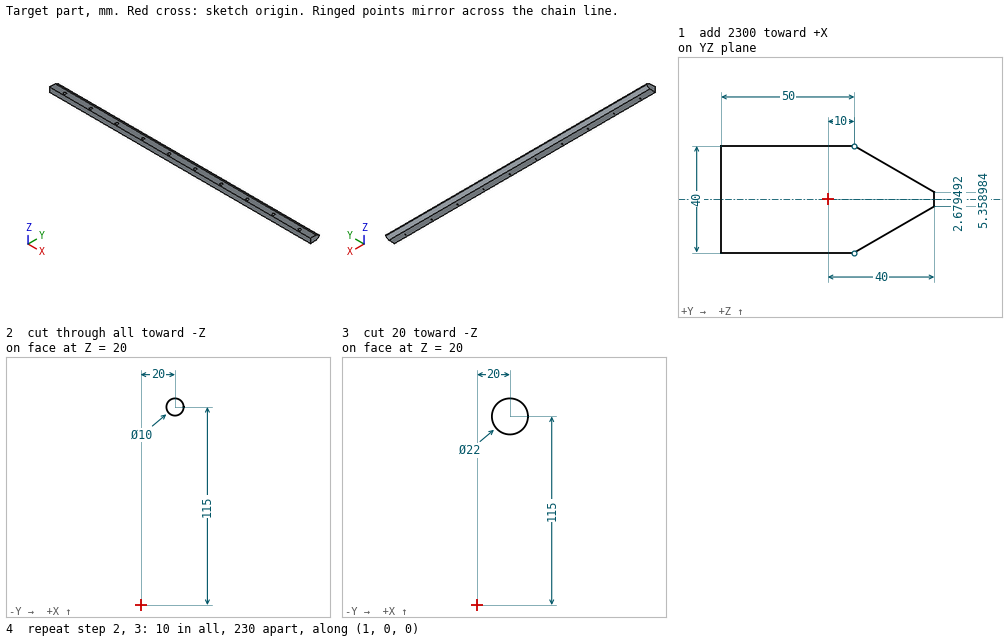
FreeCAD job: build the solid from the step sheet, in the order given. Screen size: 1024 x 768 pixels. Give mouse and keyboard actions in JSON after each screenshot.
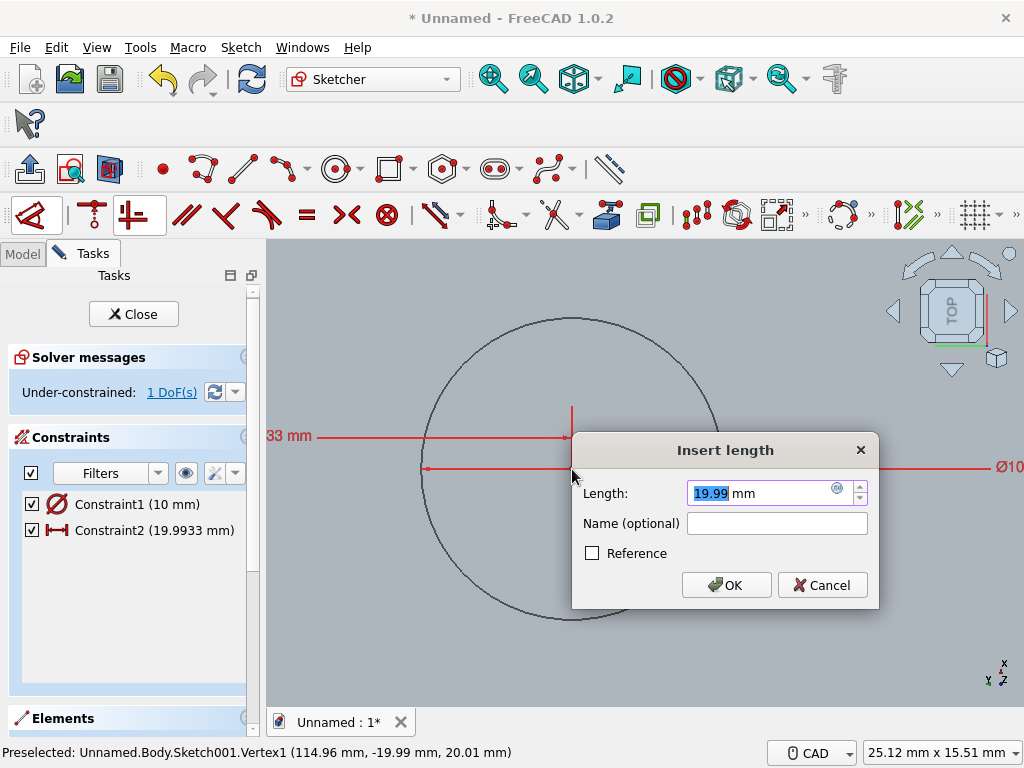
{"action": "type", "text": "20"}
{"action": "key", "text": "Return"}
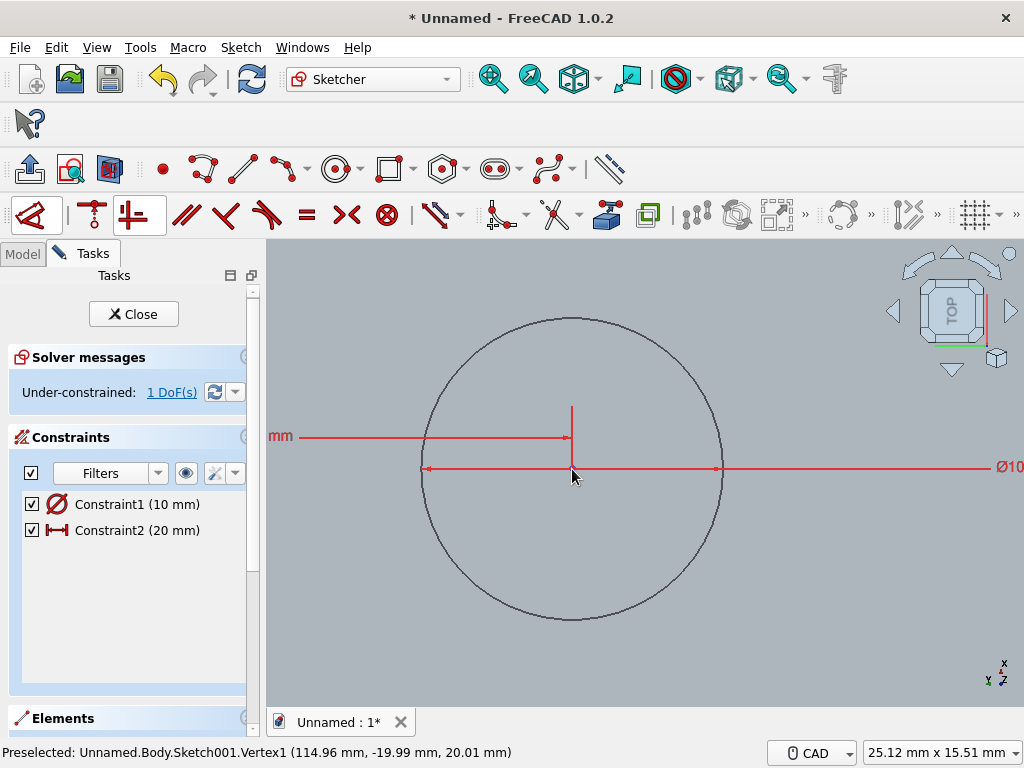
{"action": "left_click", "coordinate": [572, 469]}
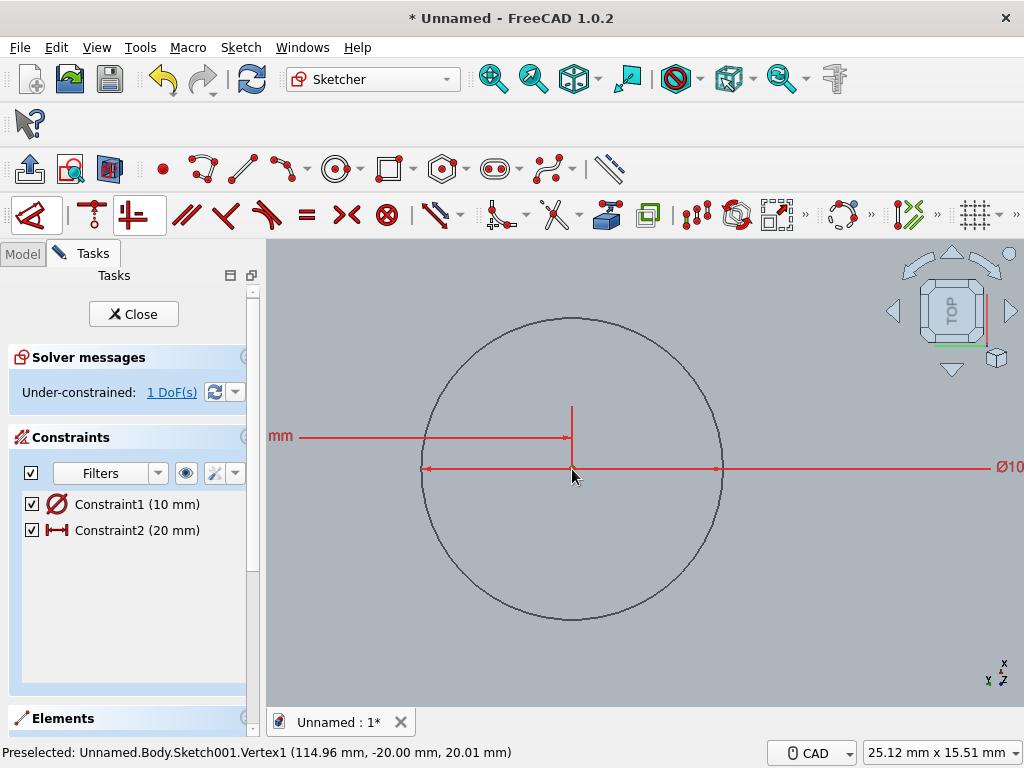
{"action": "key", "text": "i"}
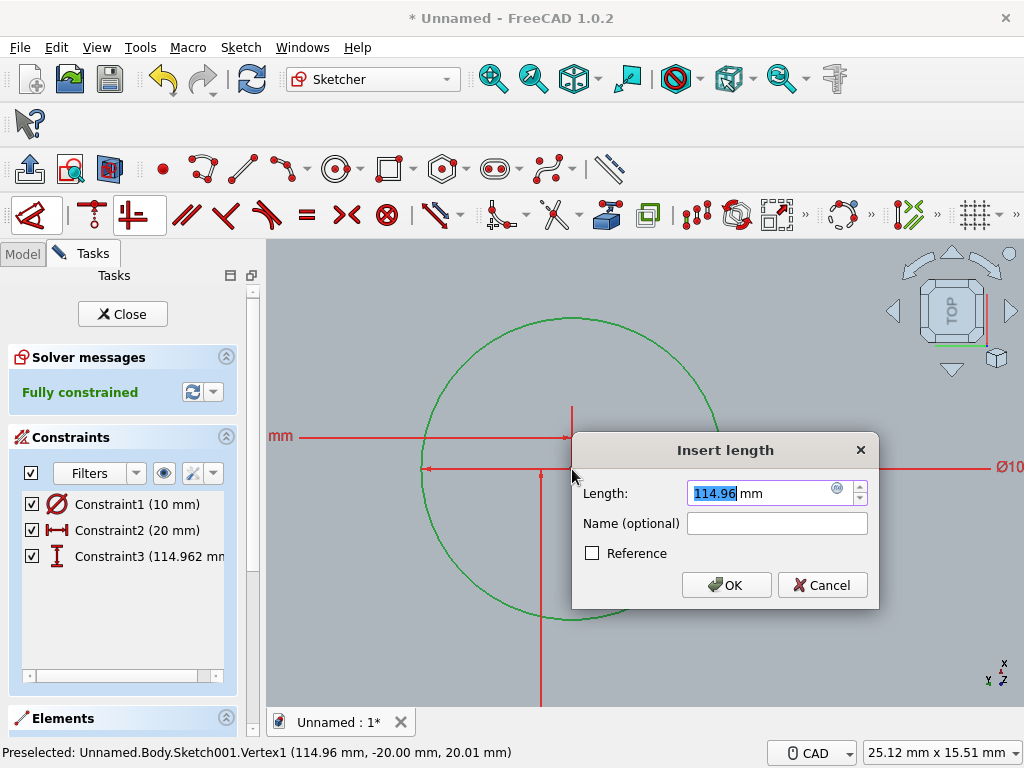
{"action": "type", "text": "115"}
{"action": "key", "text": "Return"}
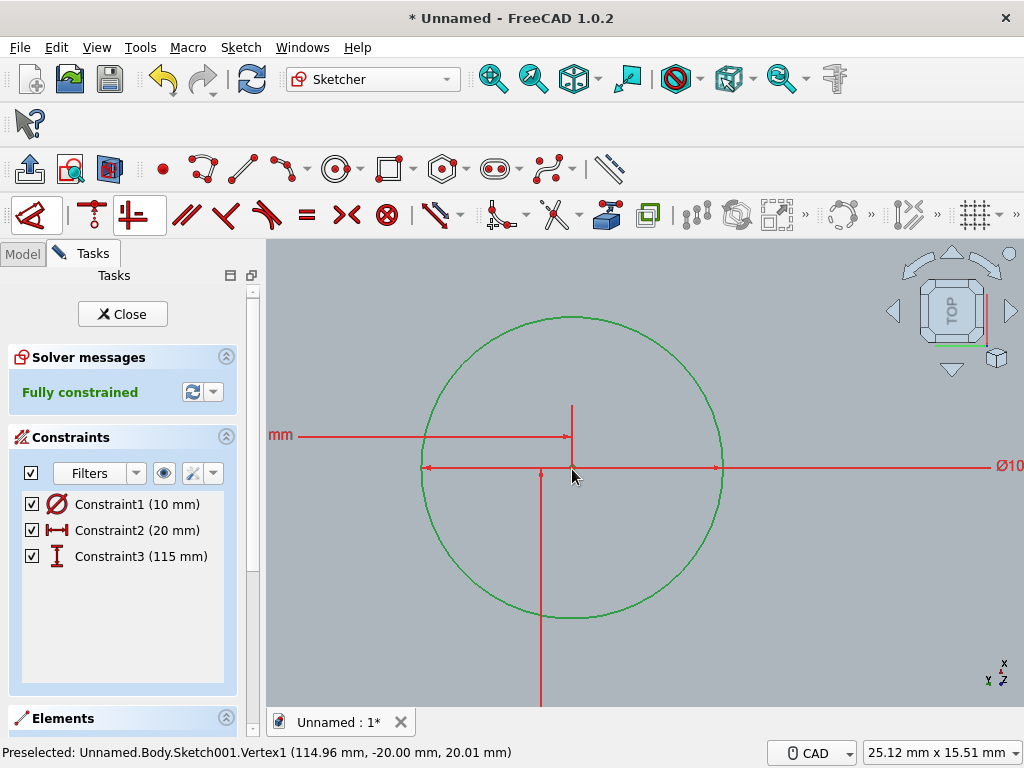
{"action": "left_click", "coordinate": [123, 314]}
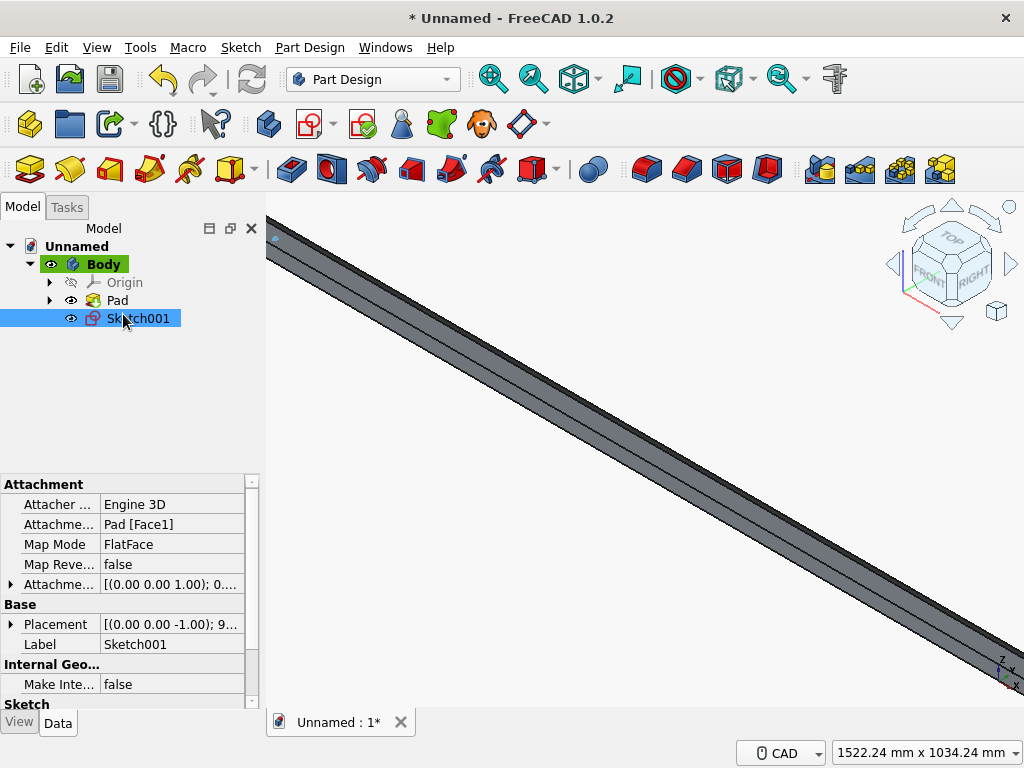
{"action": "left_click", "coordinate": [292, 170]}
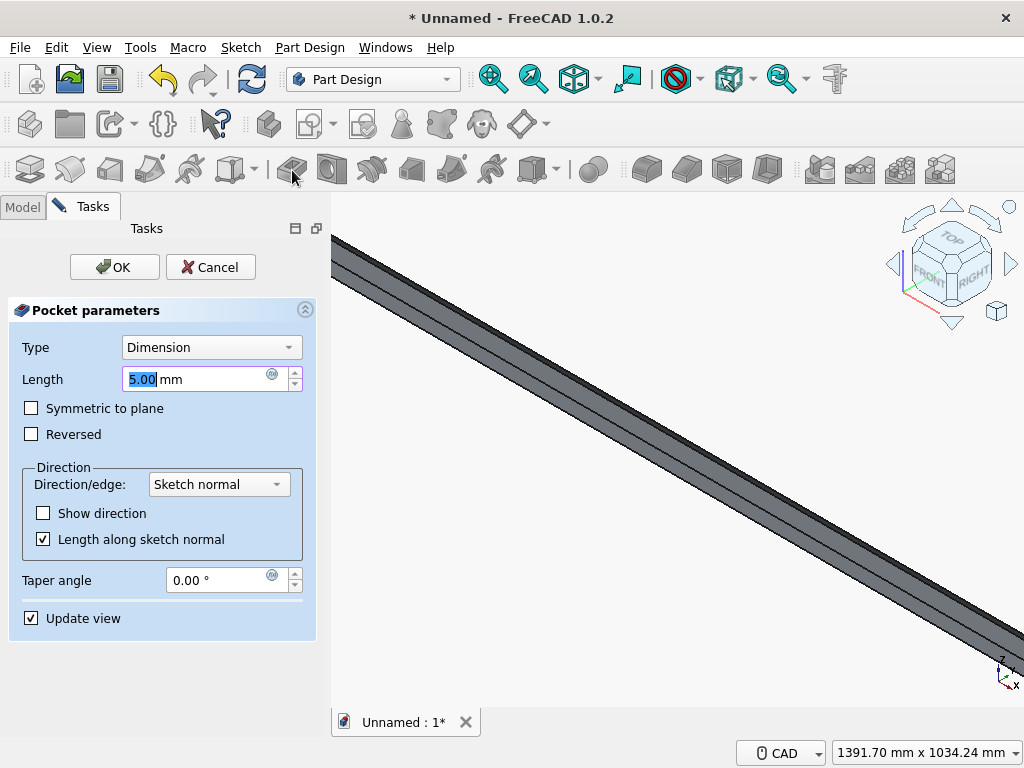
{"action": "left_click", "coordinate": [212, 348]}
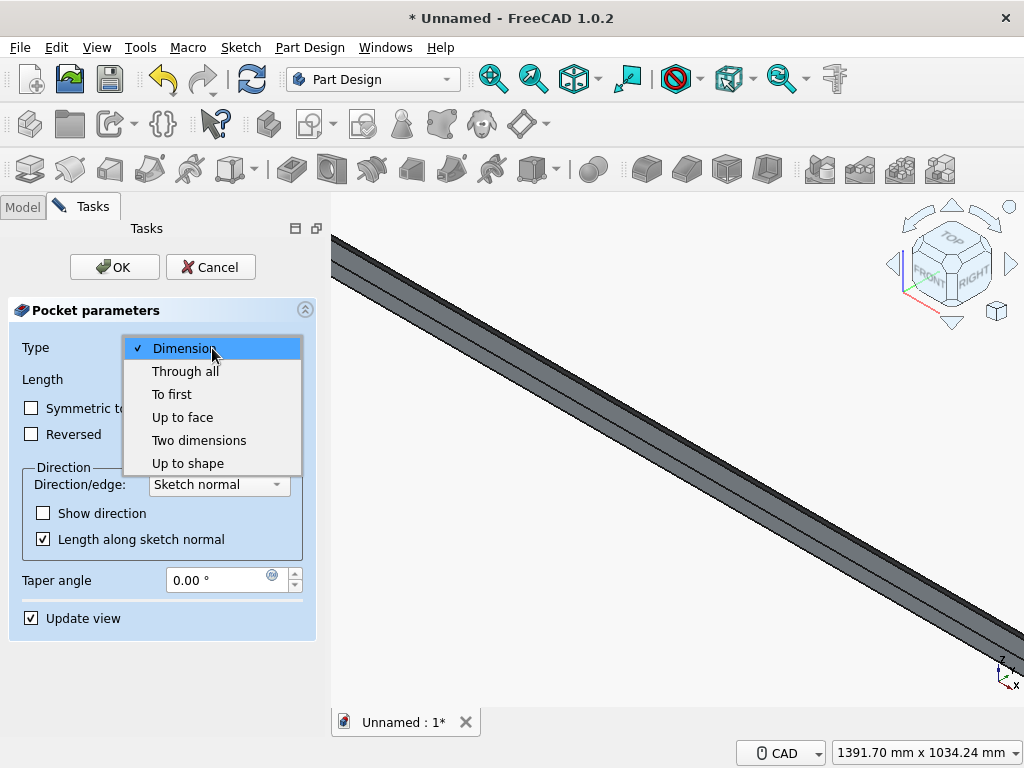
{"action": "left_click", "coordinate": [212, 372]}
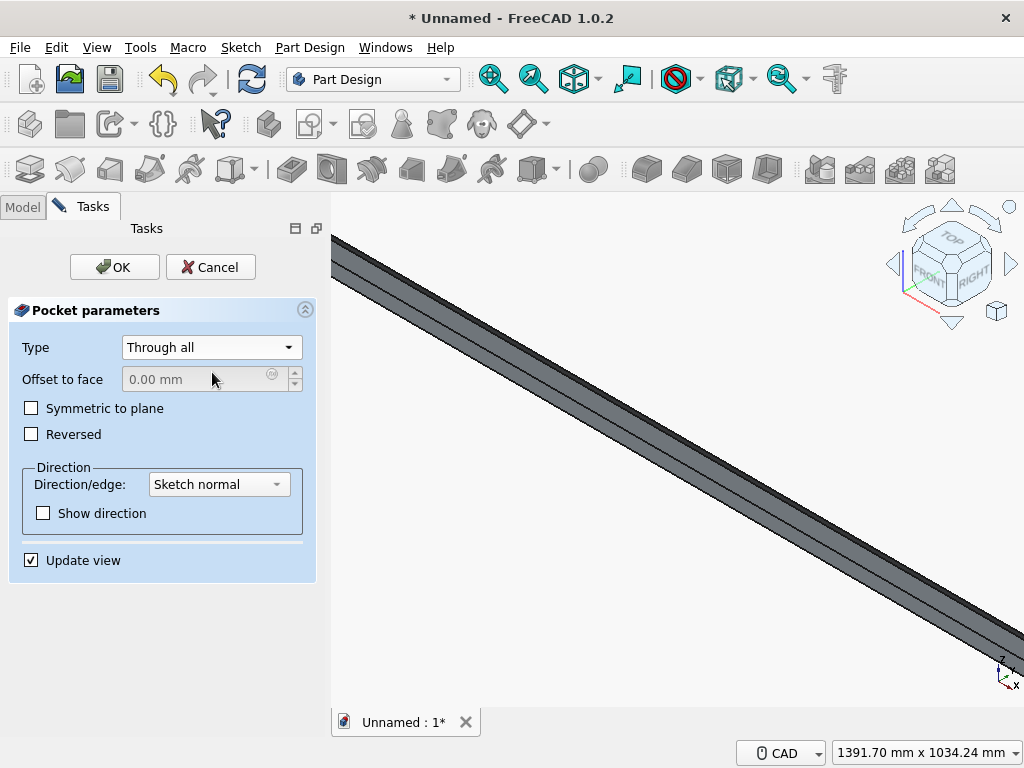
{"action": "left_click", "coordinate": [115, 267]}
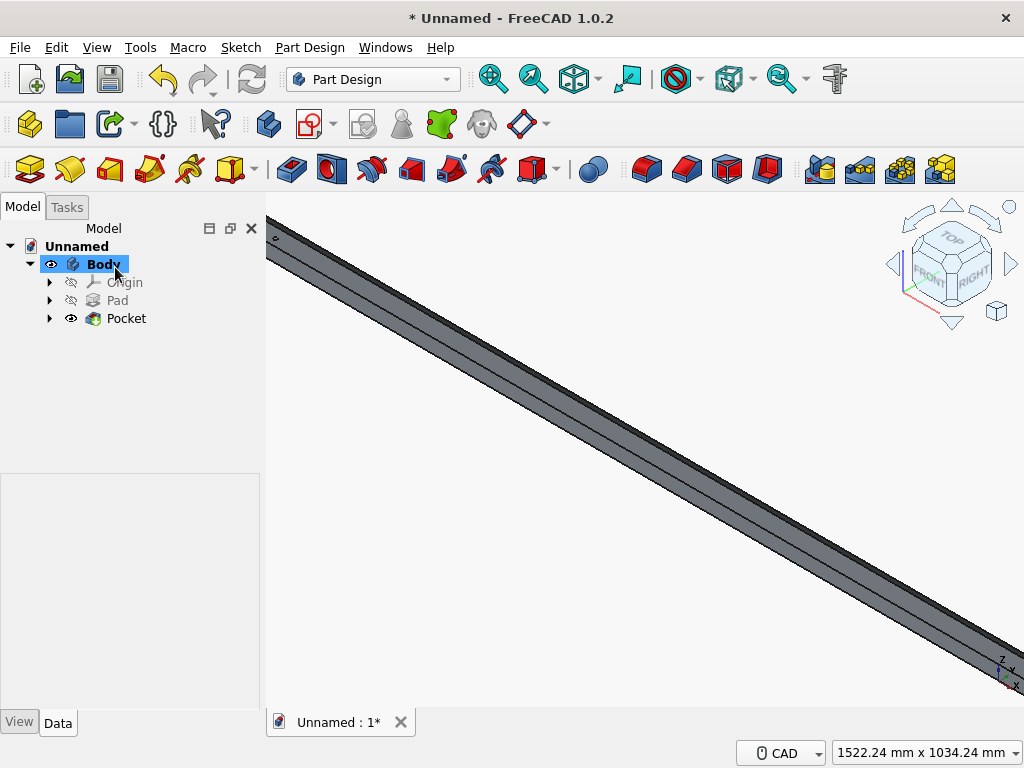
{"action": "key", "text": "v f"}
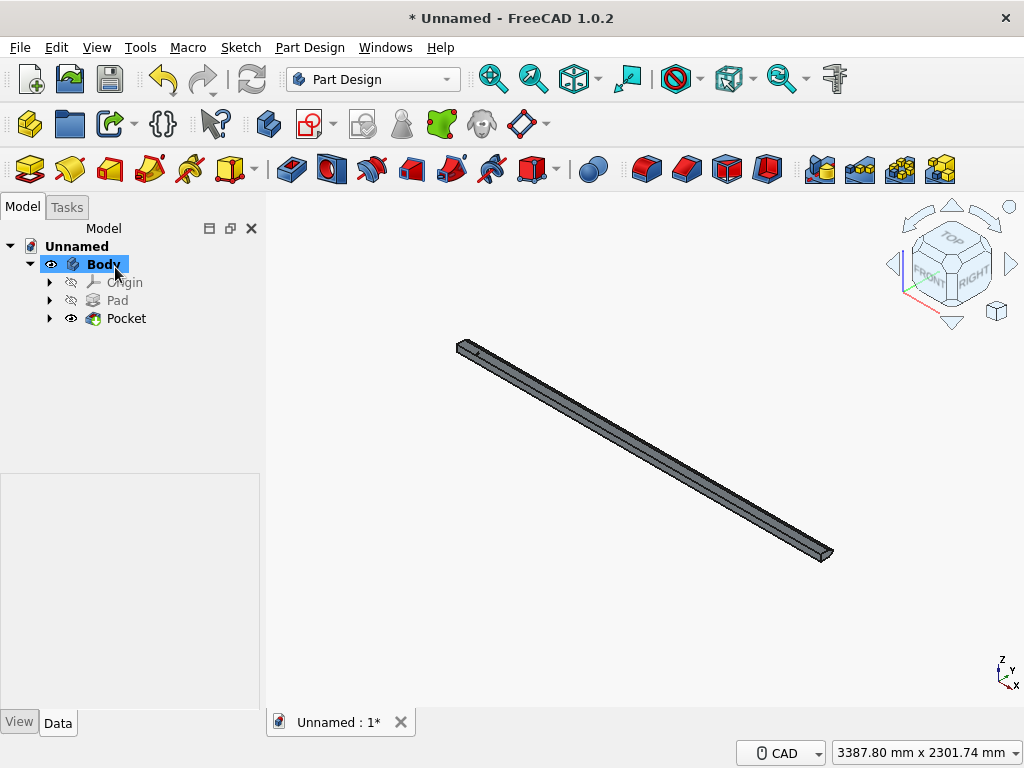
{"action": "scroll", "coordinate": [643, 446], "scroll_direction": "up", "scroll_amount": 4}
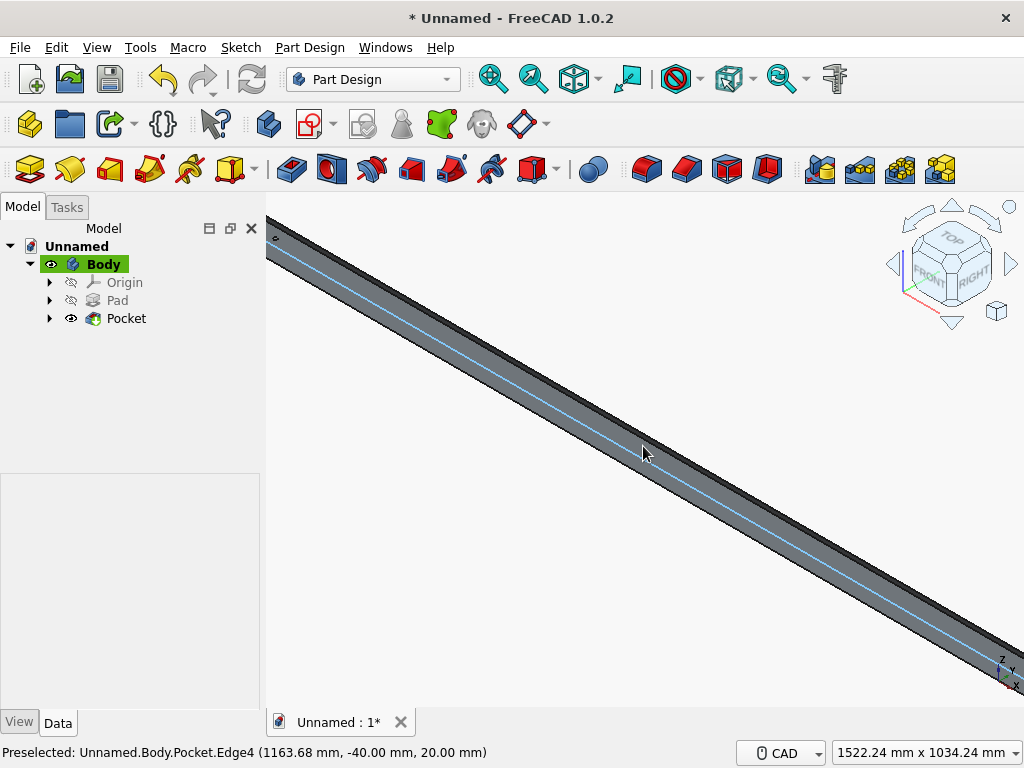
{"action": "left_click", "coordinate": [642, 447]}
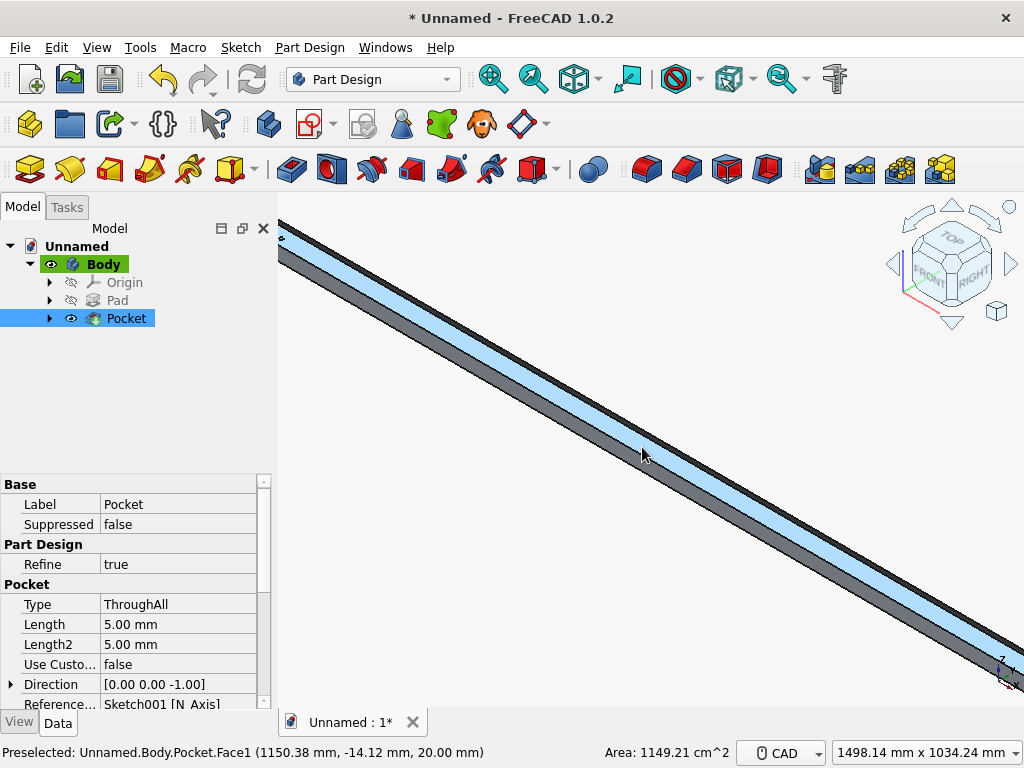
{"action": "left_click", "coordinate": [310, 124]}